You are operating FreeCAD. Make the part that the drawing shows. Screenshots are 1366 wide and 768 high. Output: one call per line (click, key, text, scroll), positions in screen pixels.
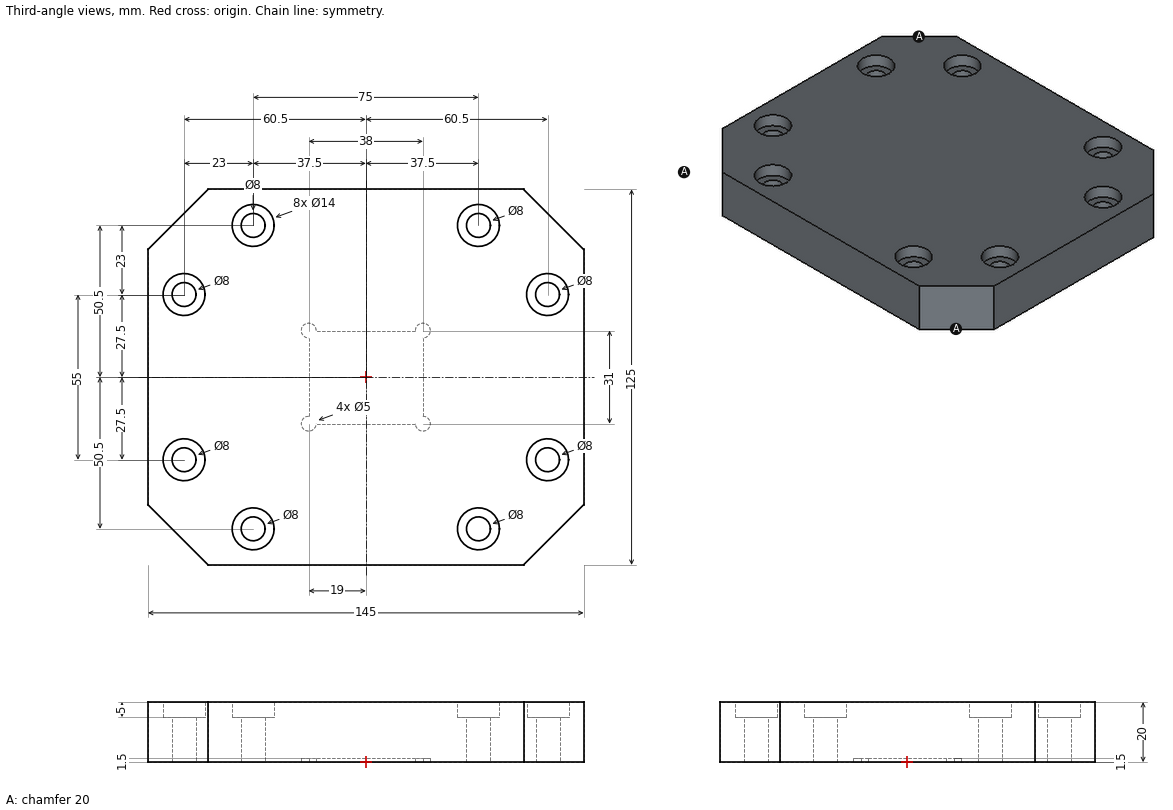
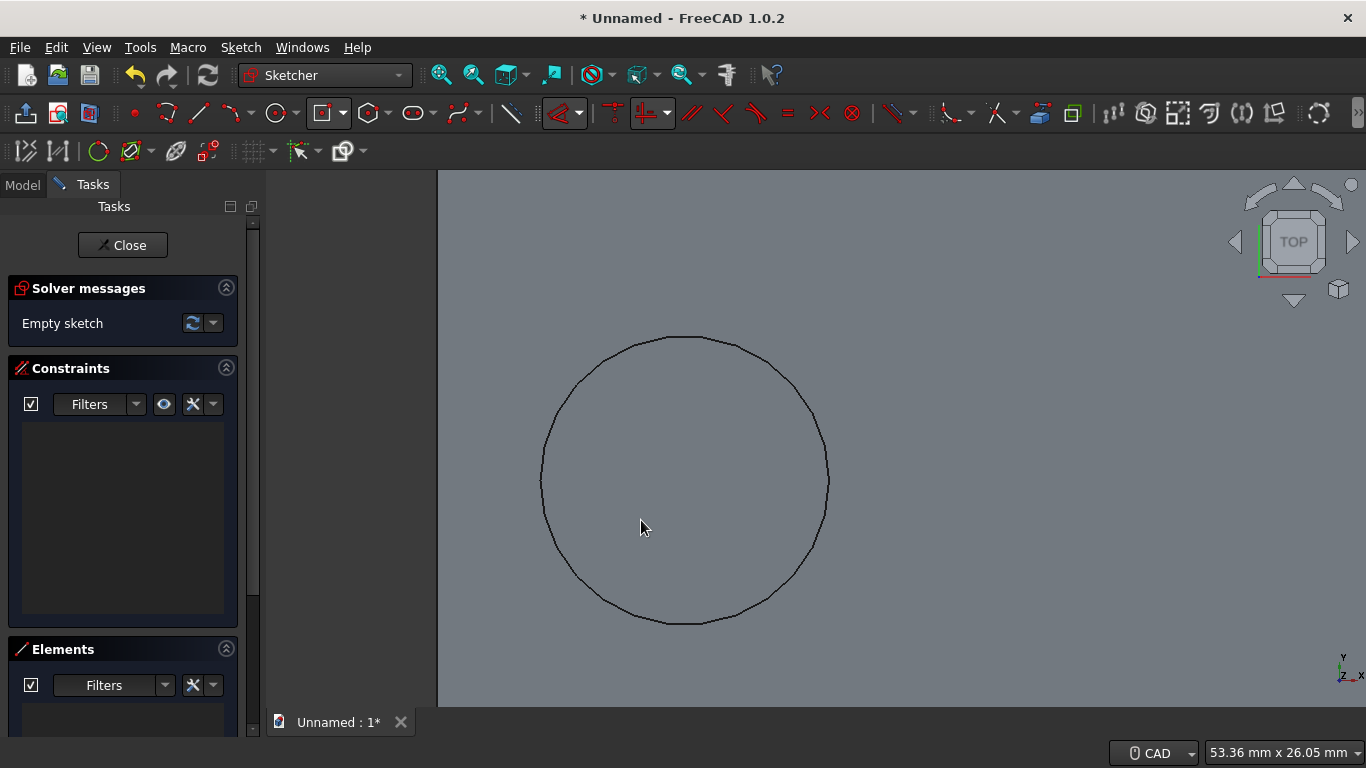
key(g)
key(c)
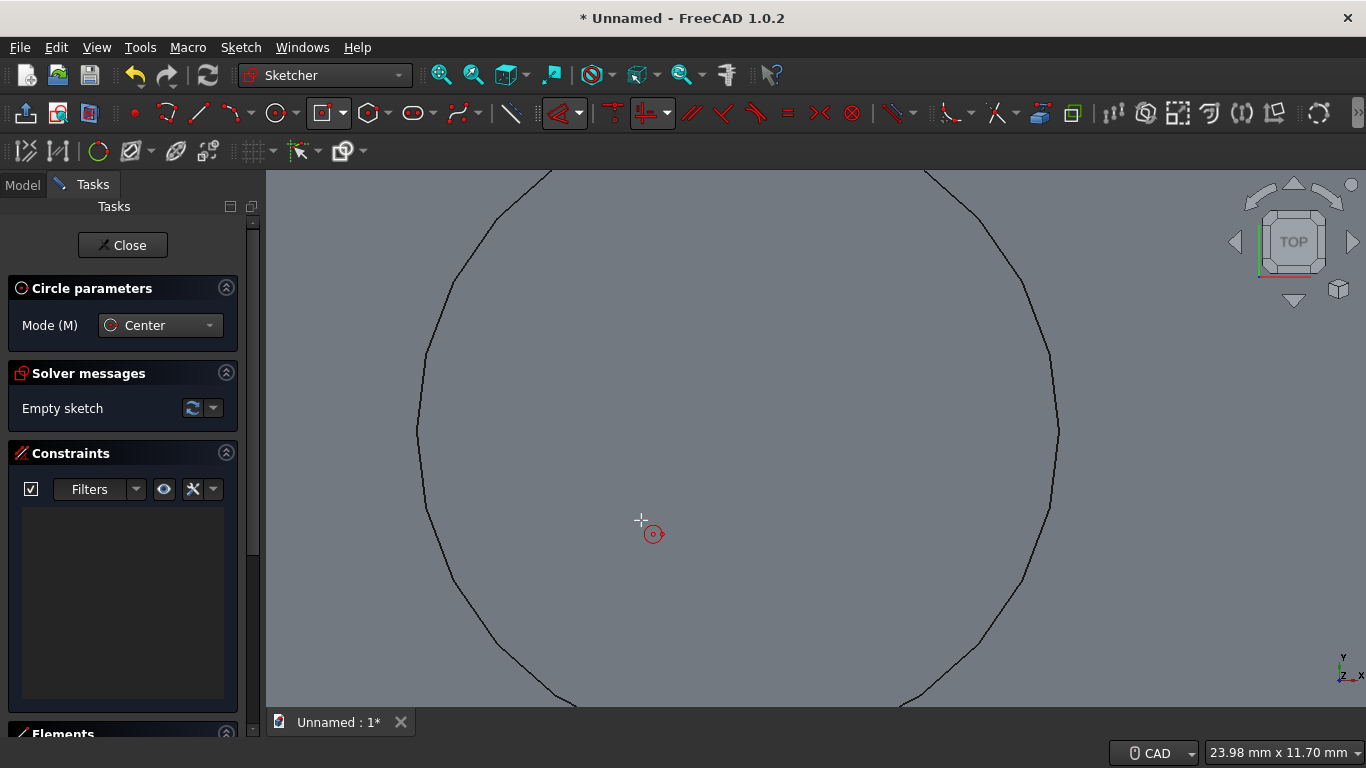
click(738, 431)
click(868, 302)
key(Escape)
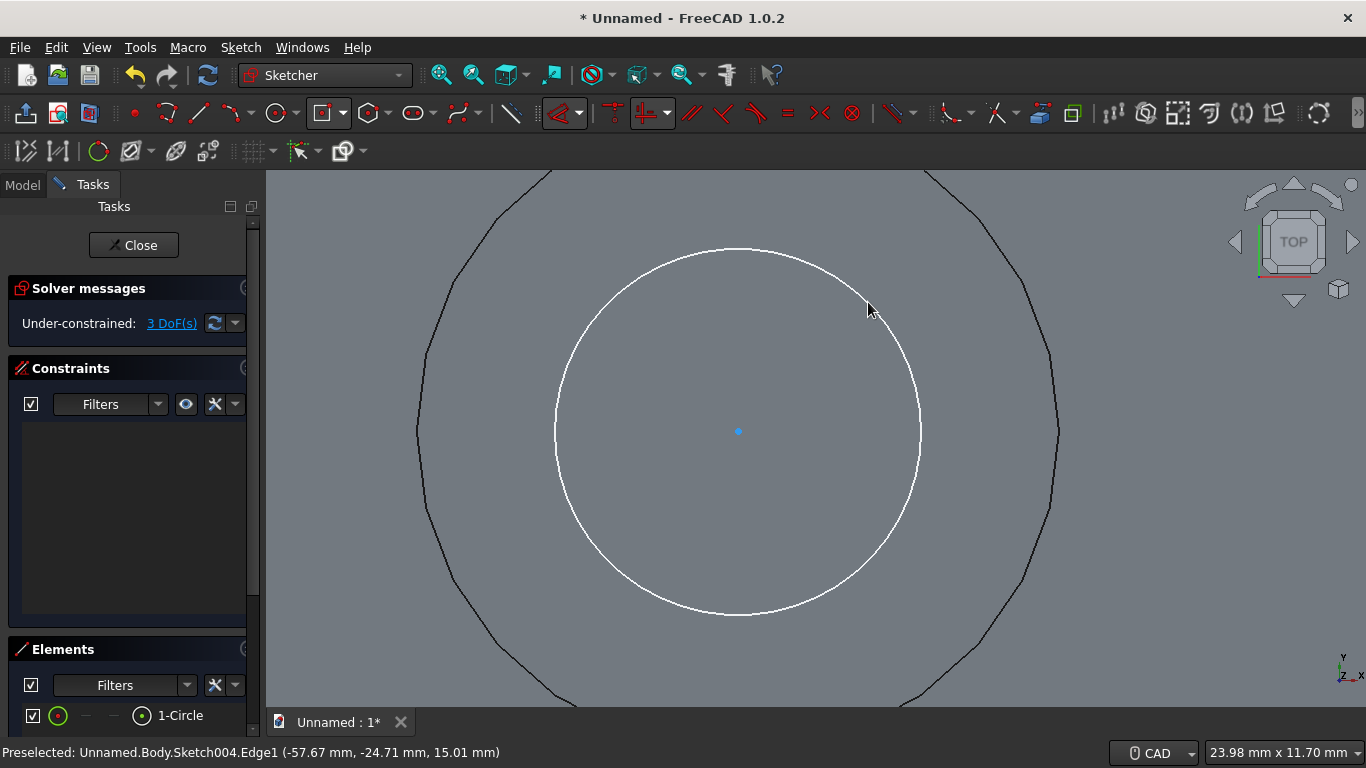
click(867, 302)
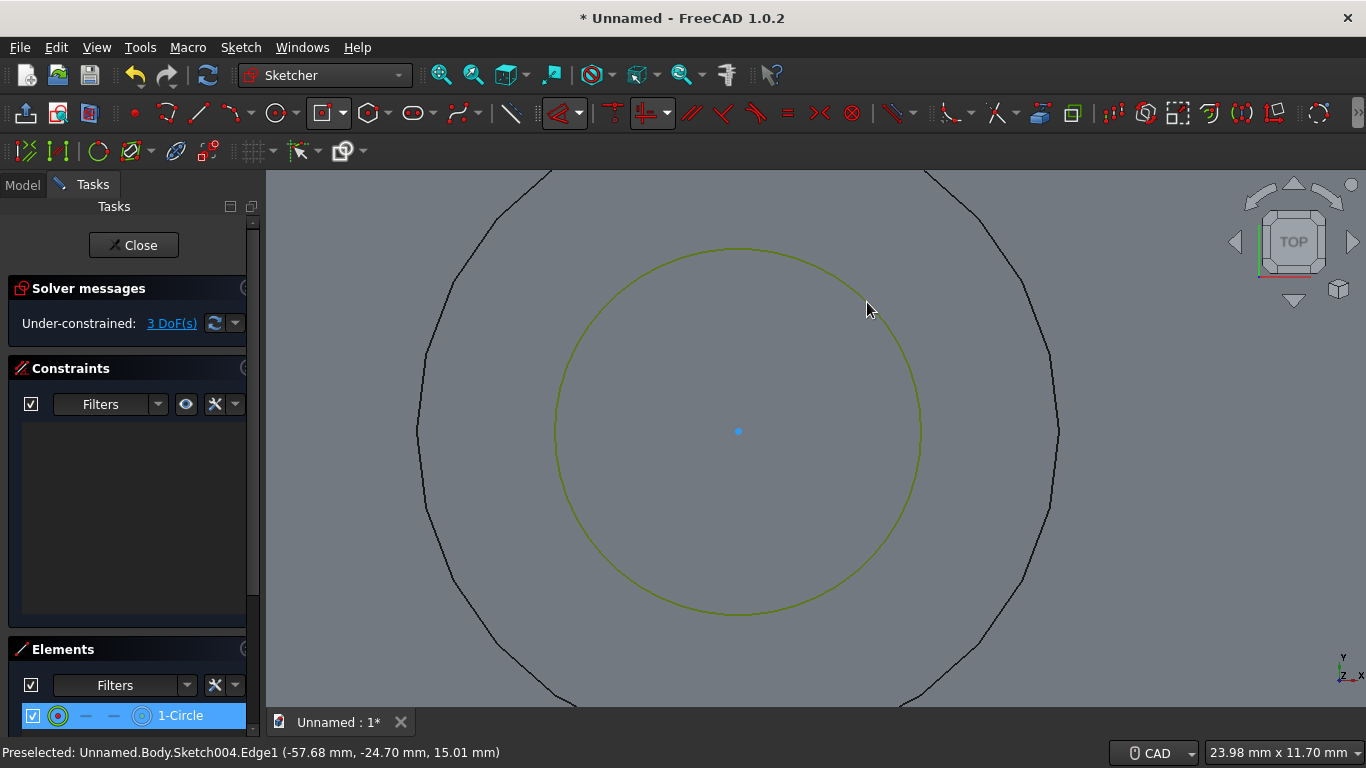
key(k)
key(o)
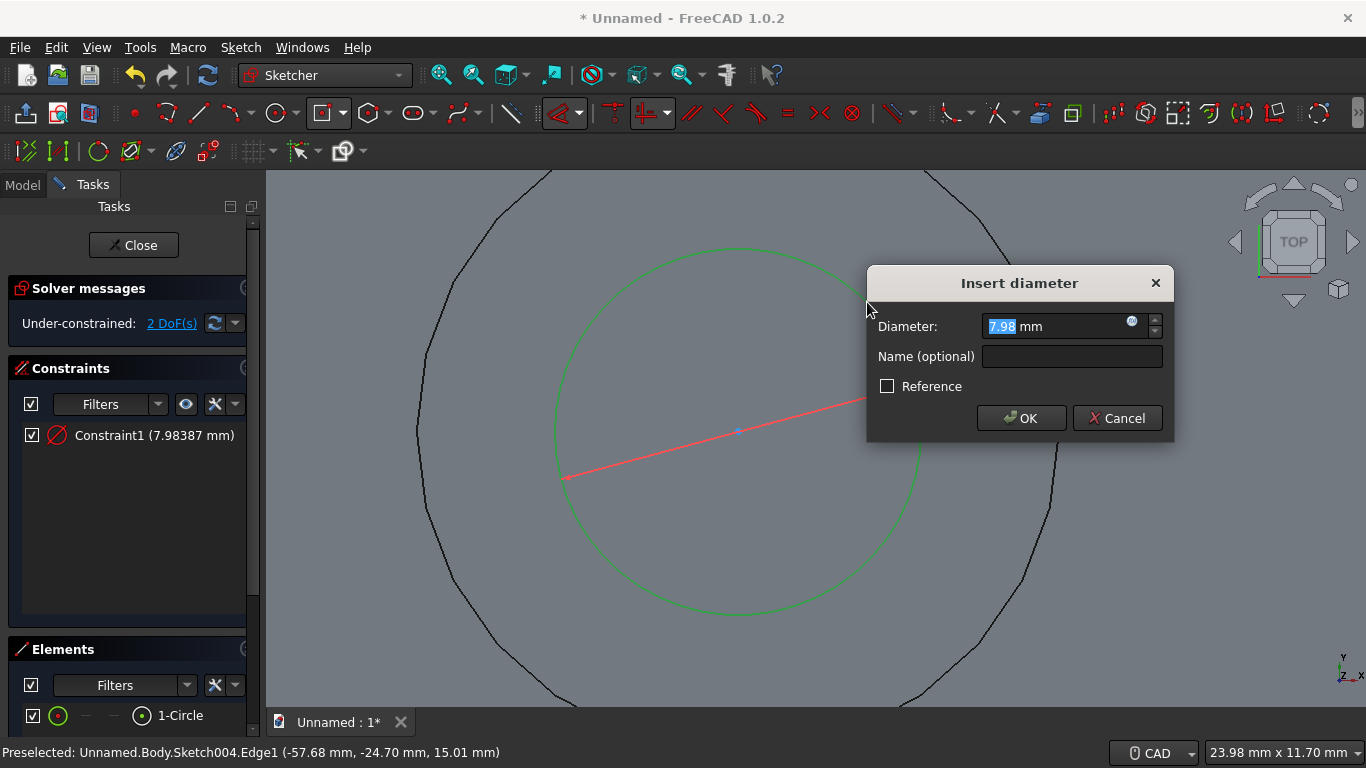
text(8)
key(Return)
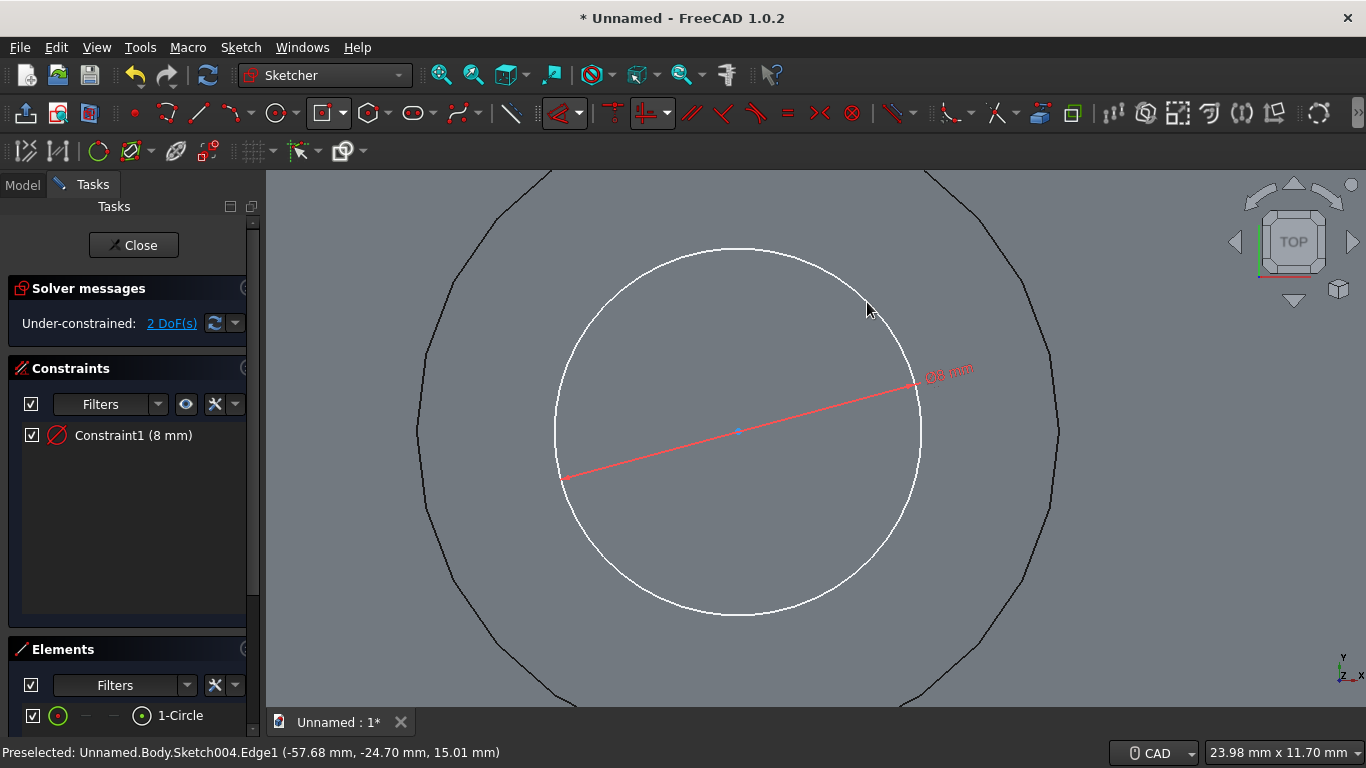
click(738, 432)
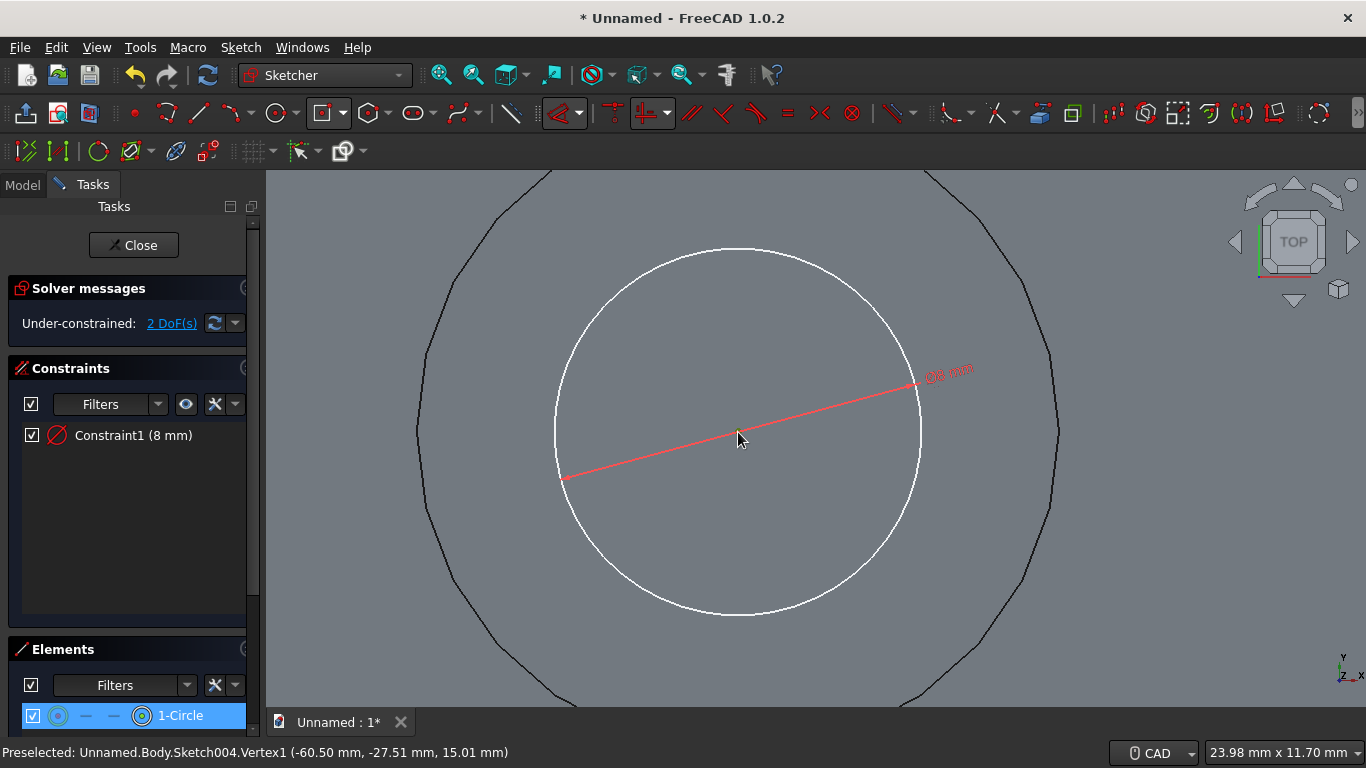
key(l)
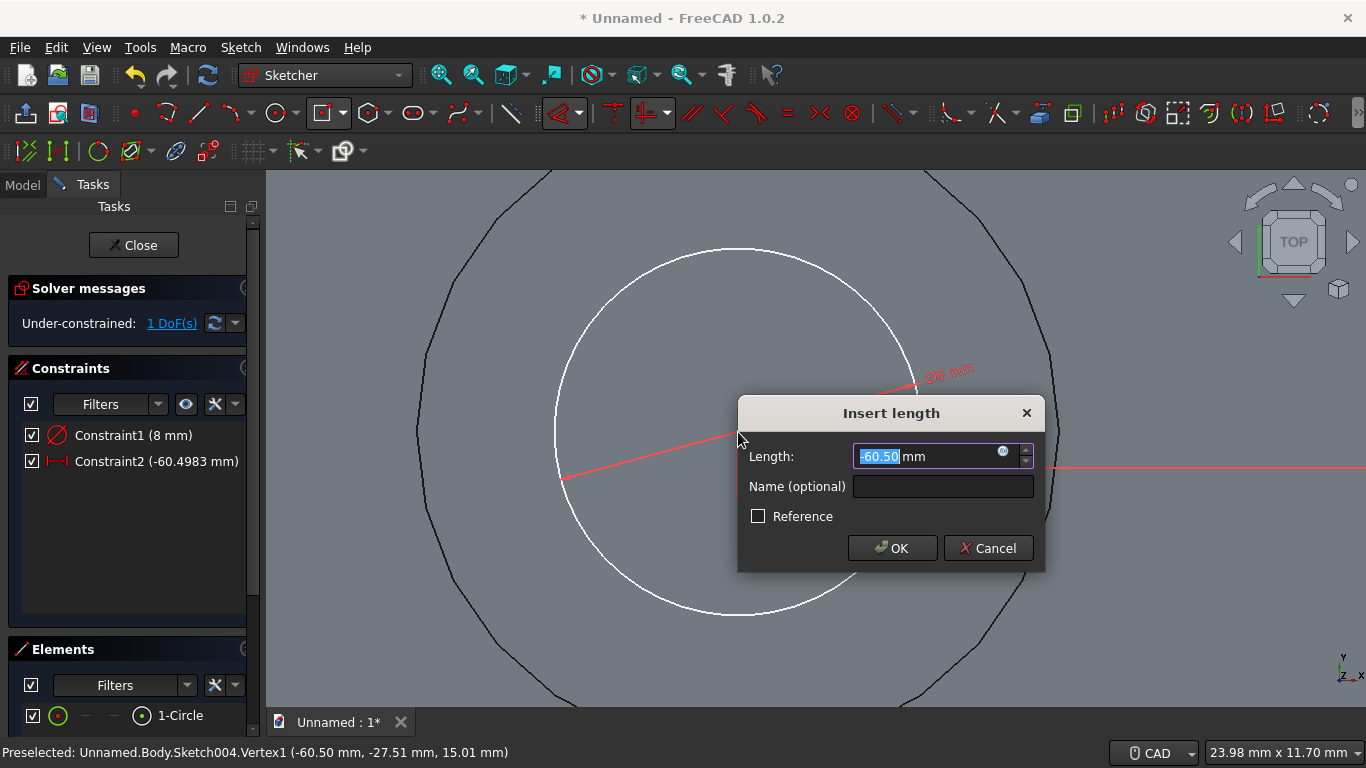
text(-60.5)
key(Return)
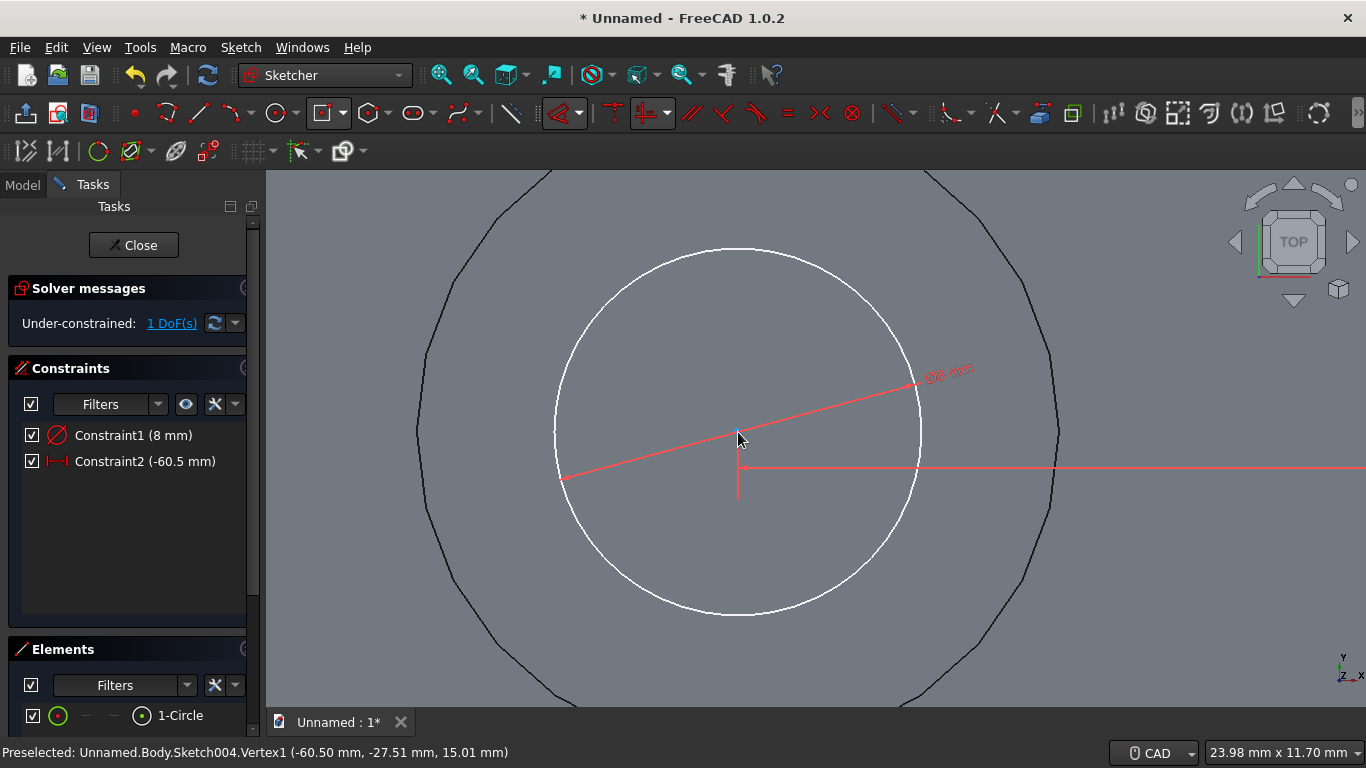
click(738, 432)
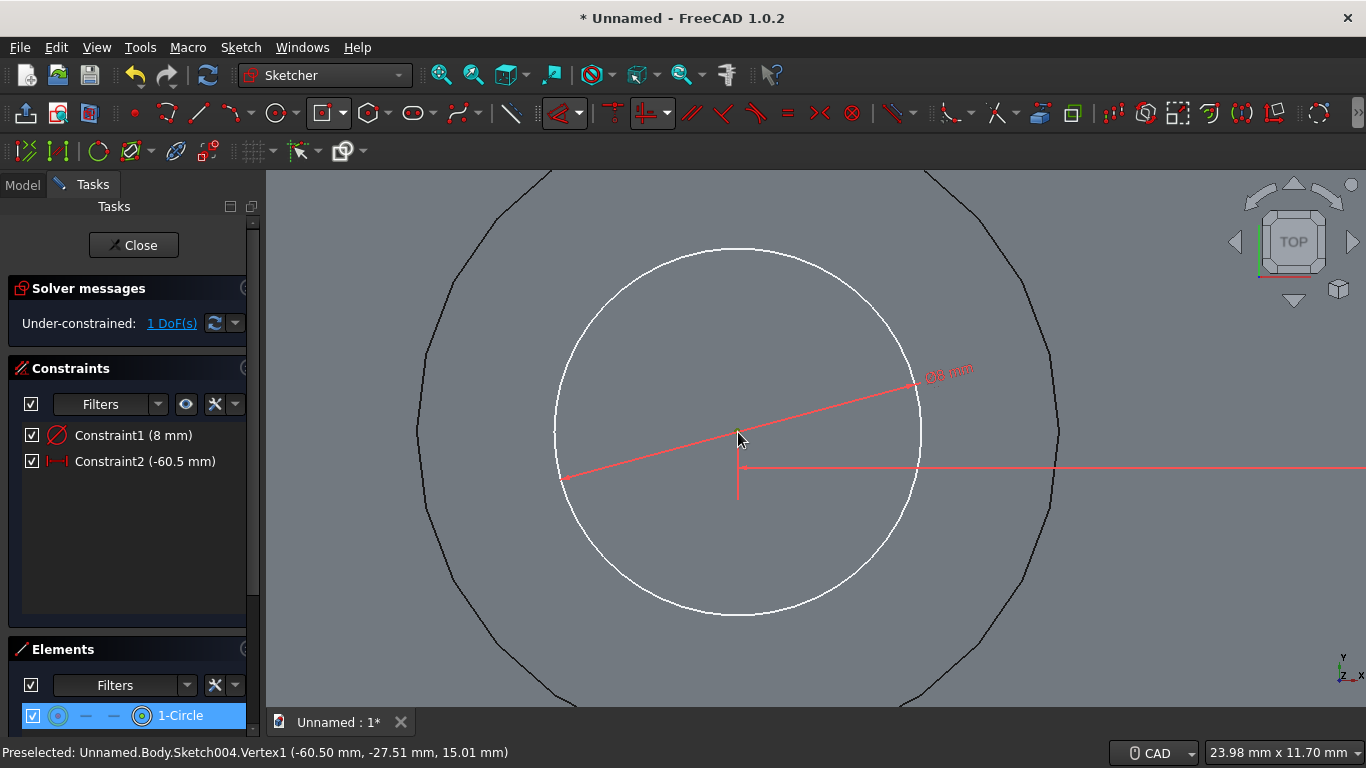
key(i)